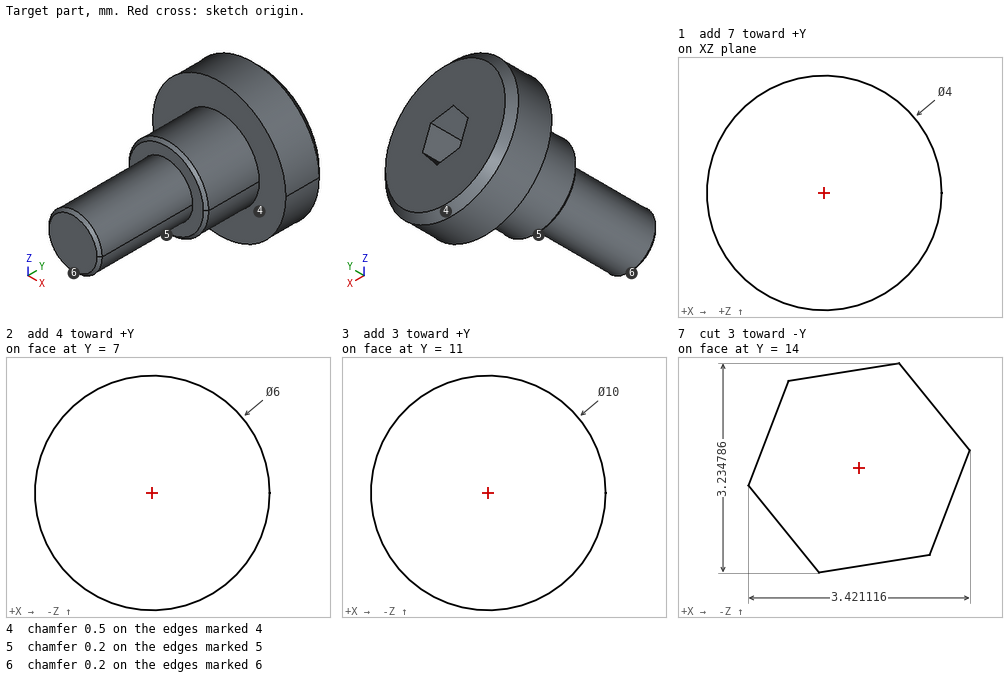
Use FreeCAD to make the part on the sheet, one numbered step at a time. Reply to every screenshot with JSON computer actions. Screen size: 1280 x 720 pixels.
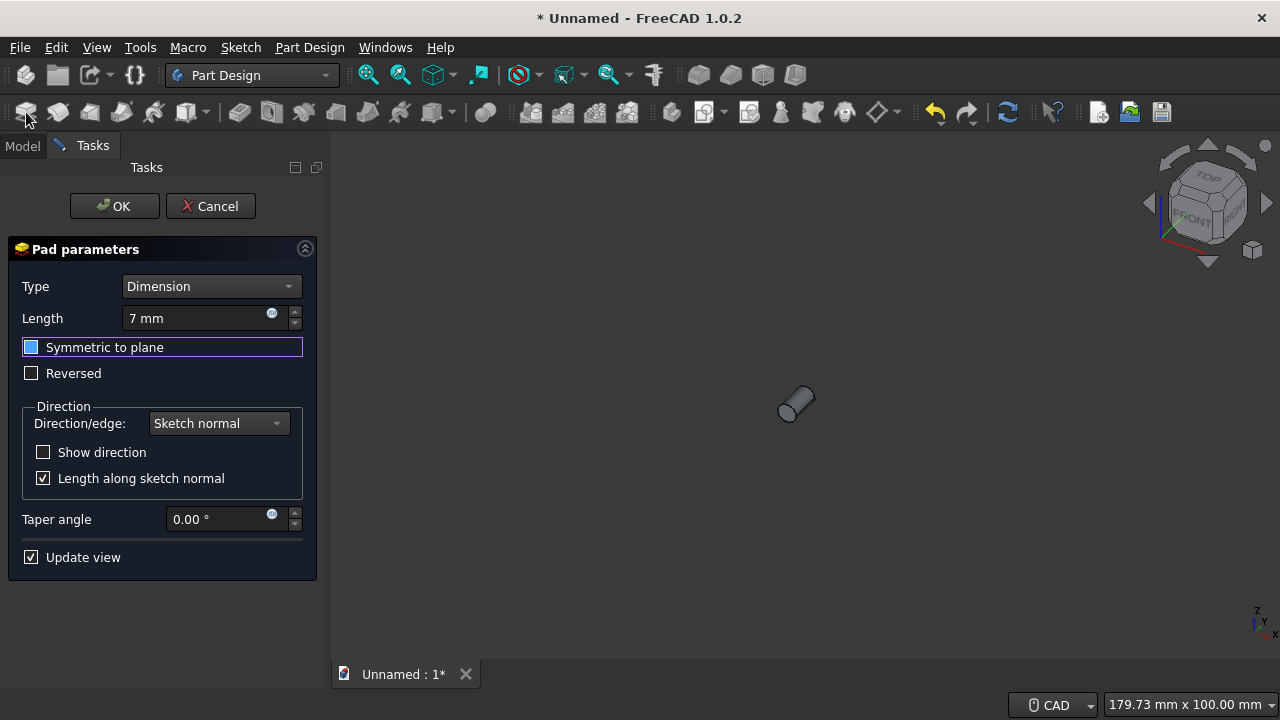
{"action": "left_click", "coordinate": [30, 373]}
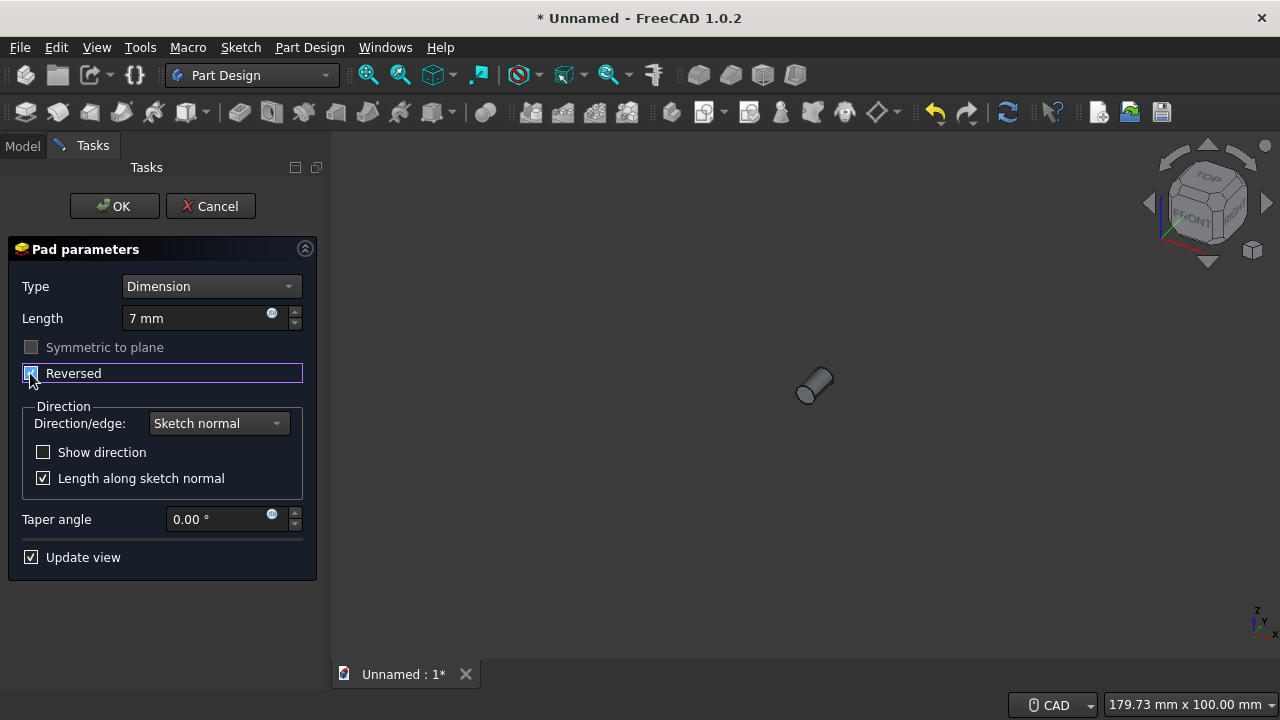
{"action": "left_click", "coordinate": [115, 206]}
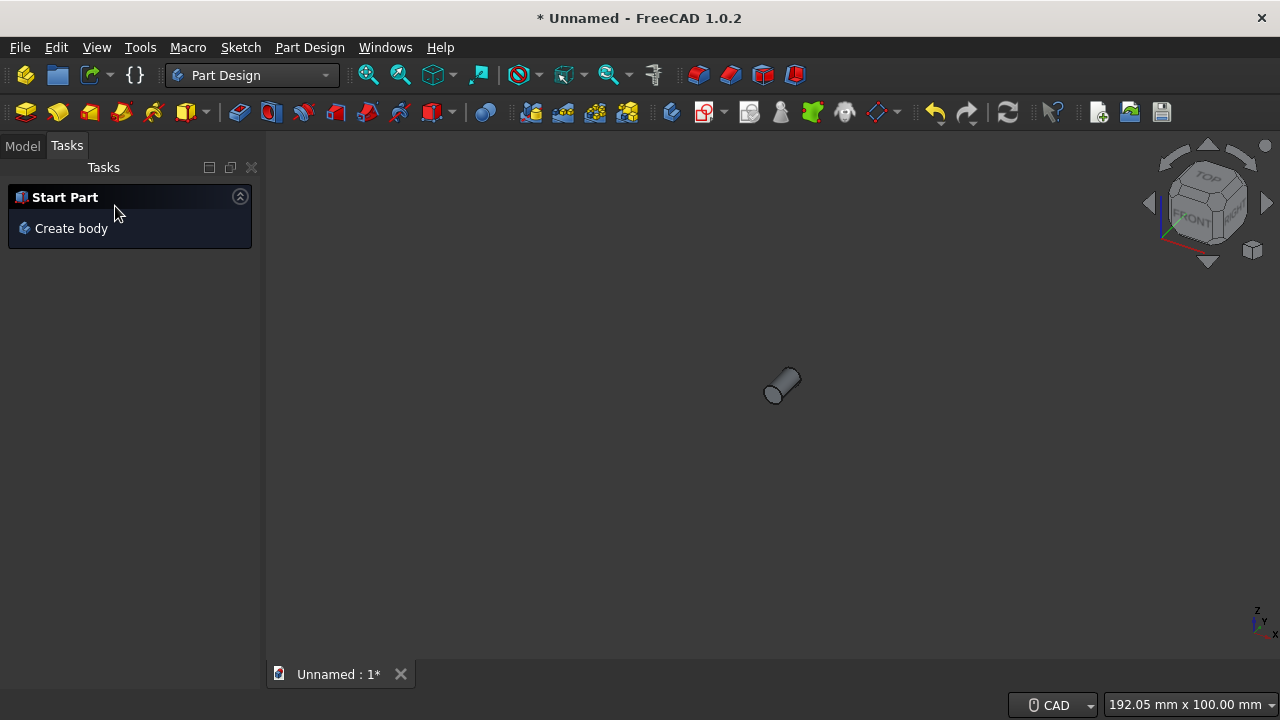
{"action": "key", "text": "v f"}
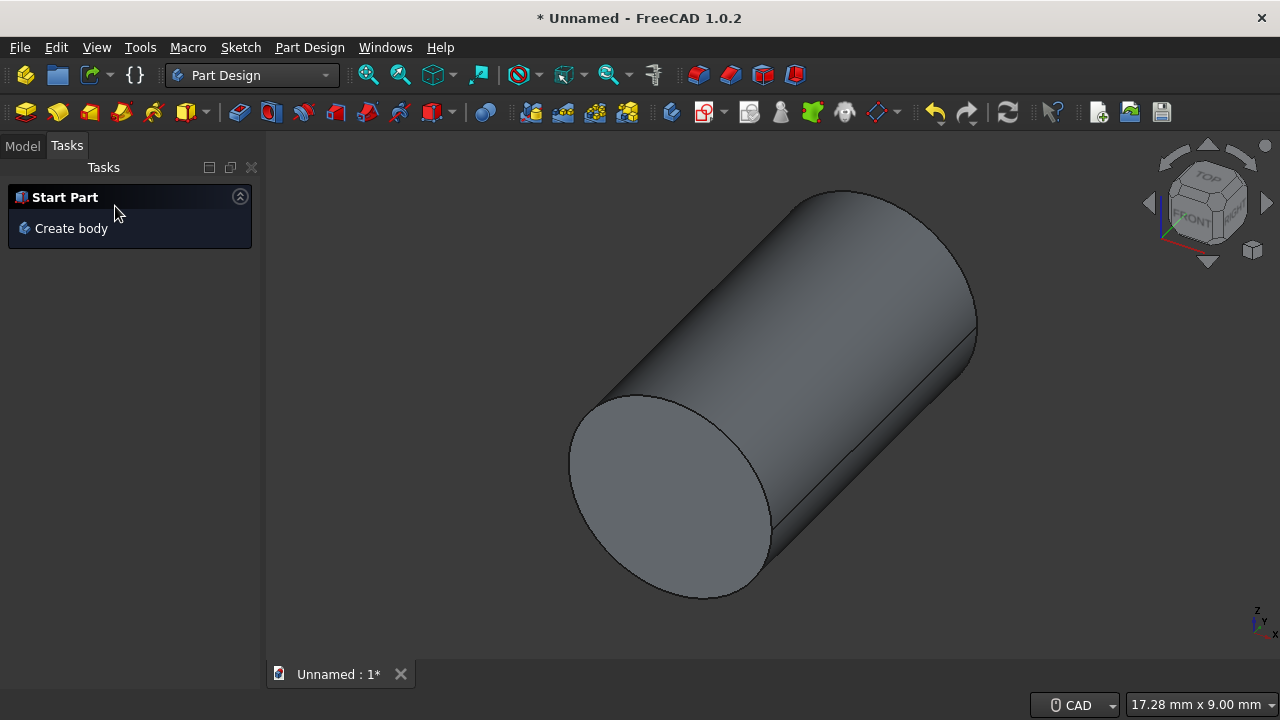
{"action": "key", "text": "4"}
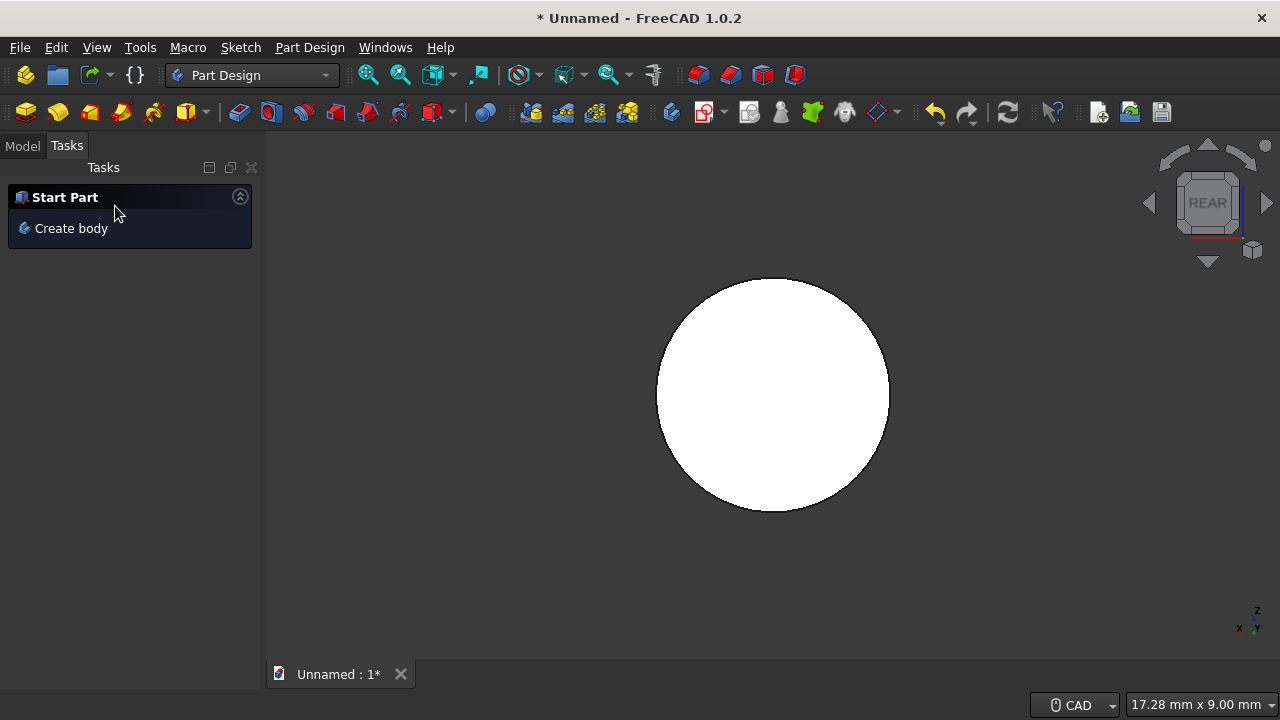
{"action": "left_click", "coordinate": [370, 76]}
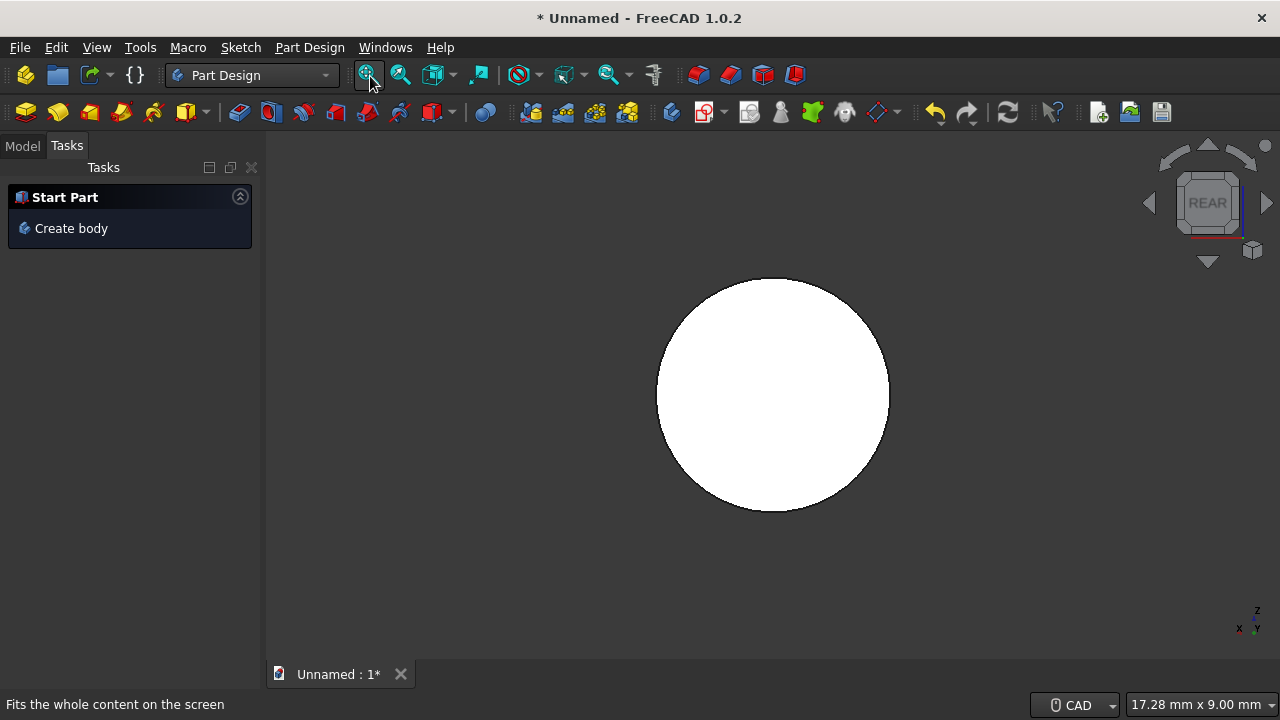
{"action": "left_click", "coordinate": [773, 394]}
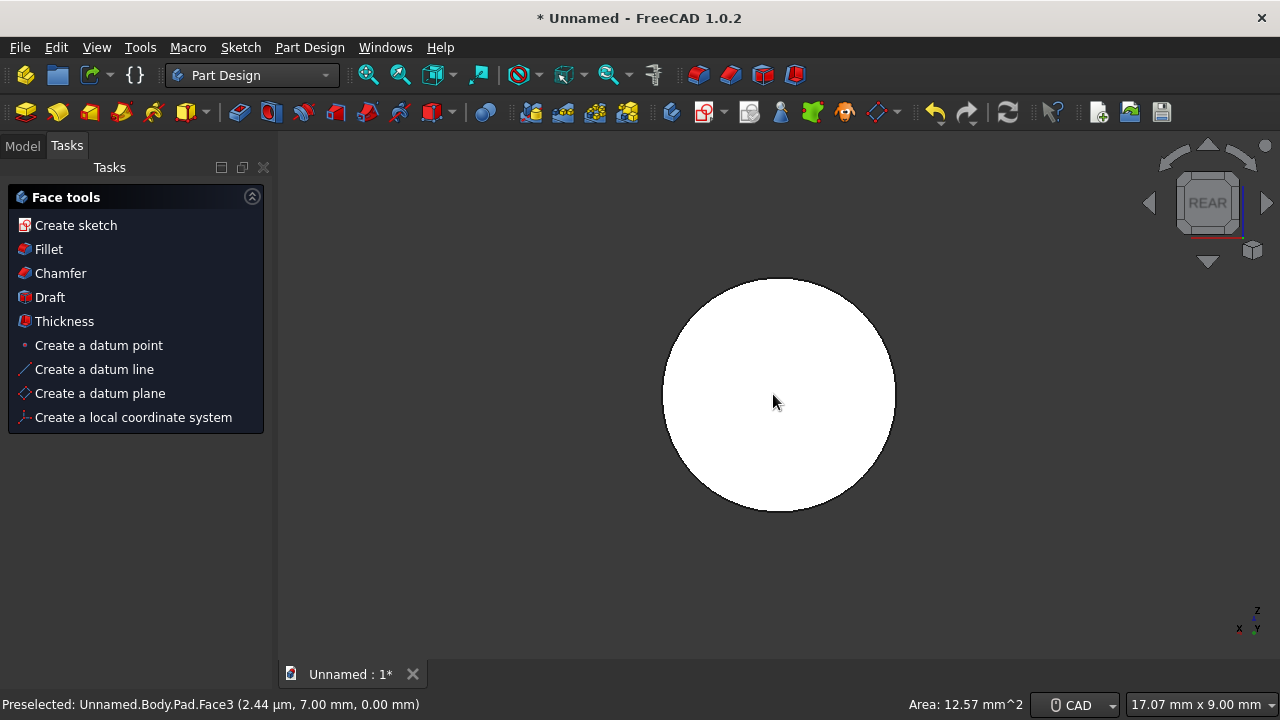
{"action": "left_click", "coordinate": [704, 112]}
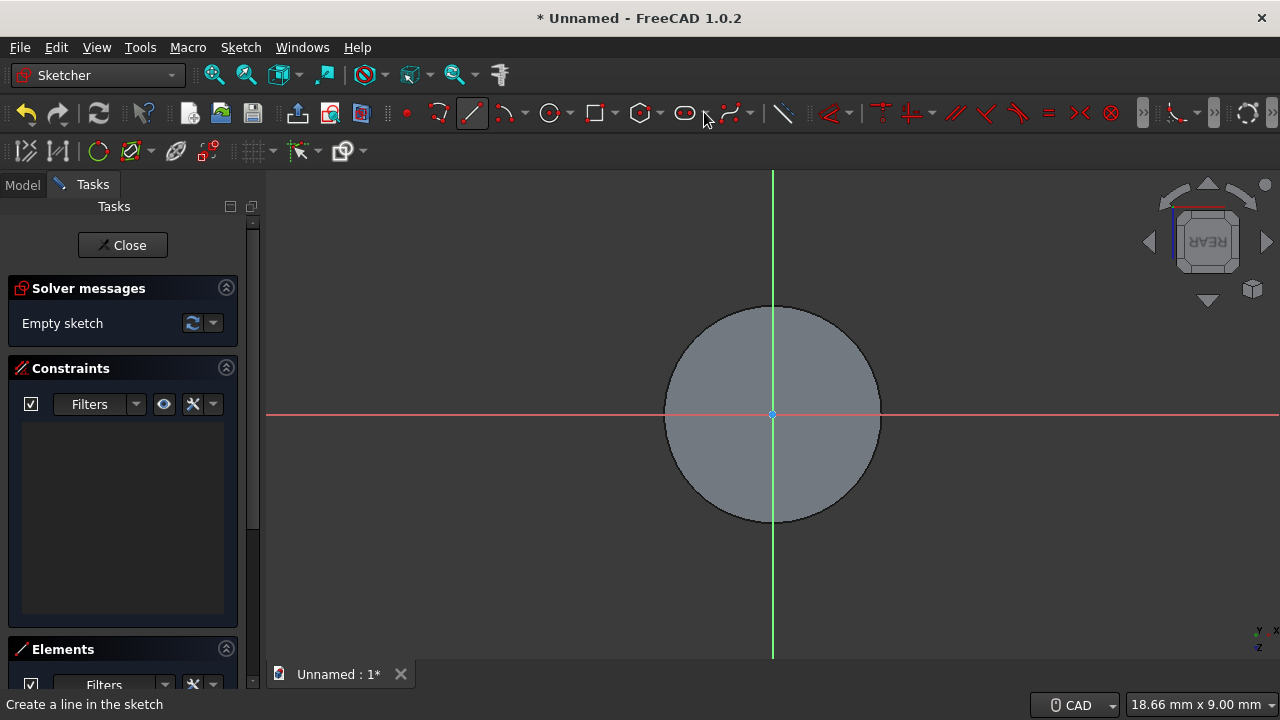
{"action": "key", "text": "g c"}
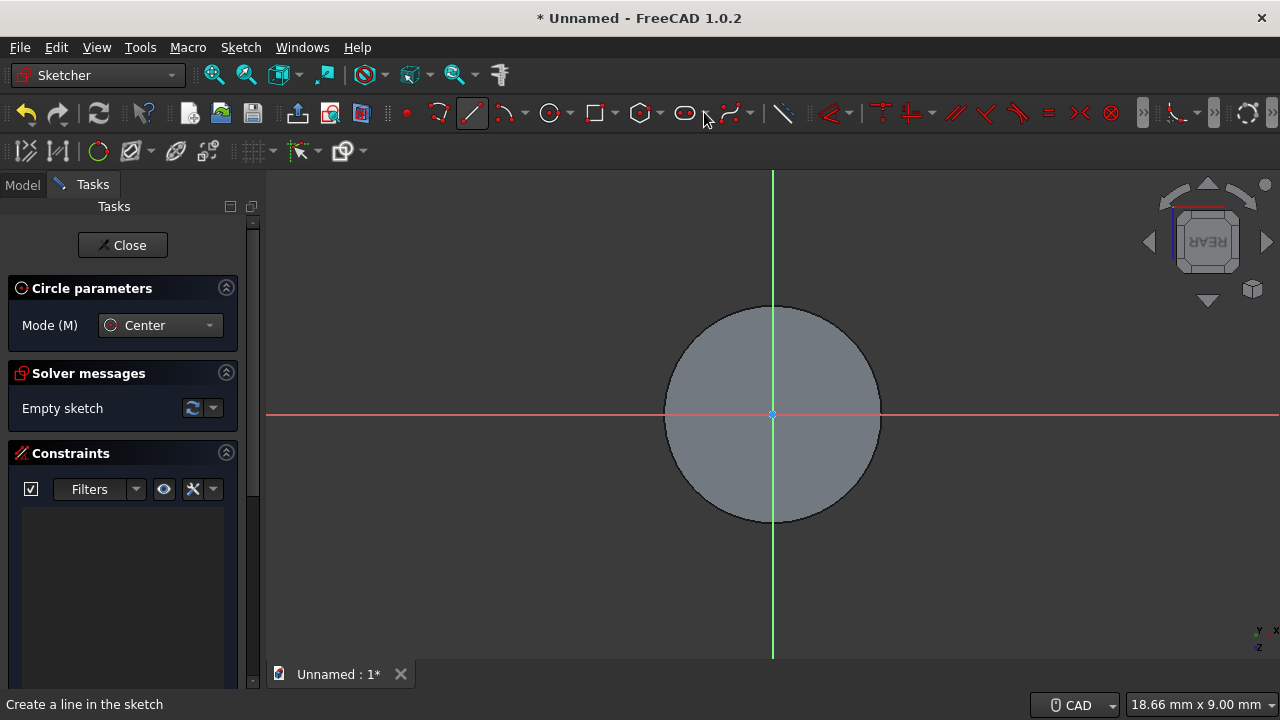
{"action": "left_click", "coordinate": [773, 414]}
{"action": "mouse_move", "coordinate": [888, 299]}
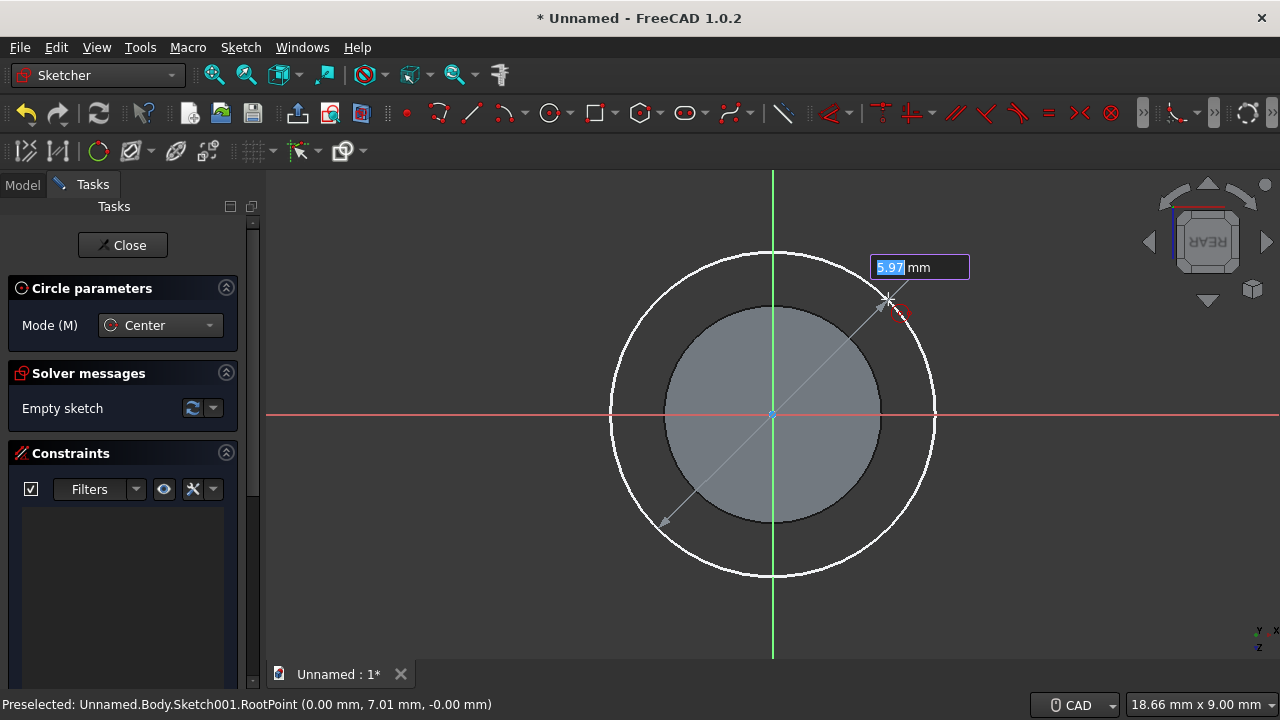
{"action": "type", "text": "6"}
{"action": "key", "text": "Return"}
{"action": "key", "text": "Escape"}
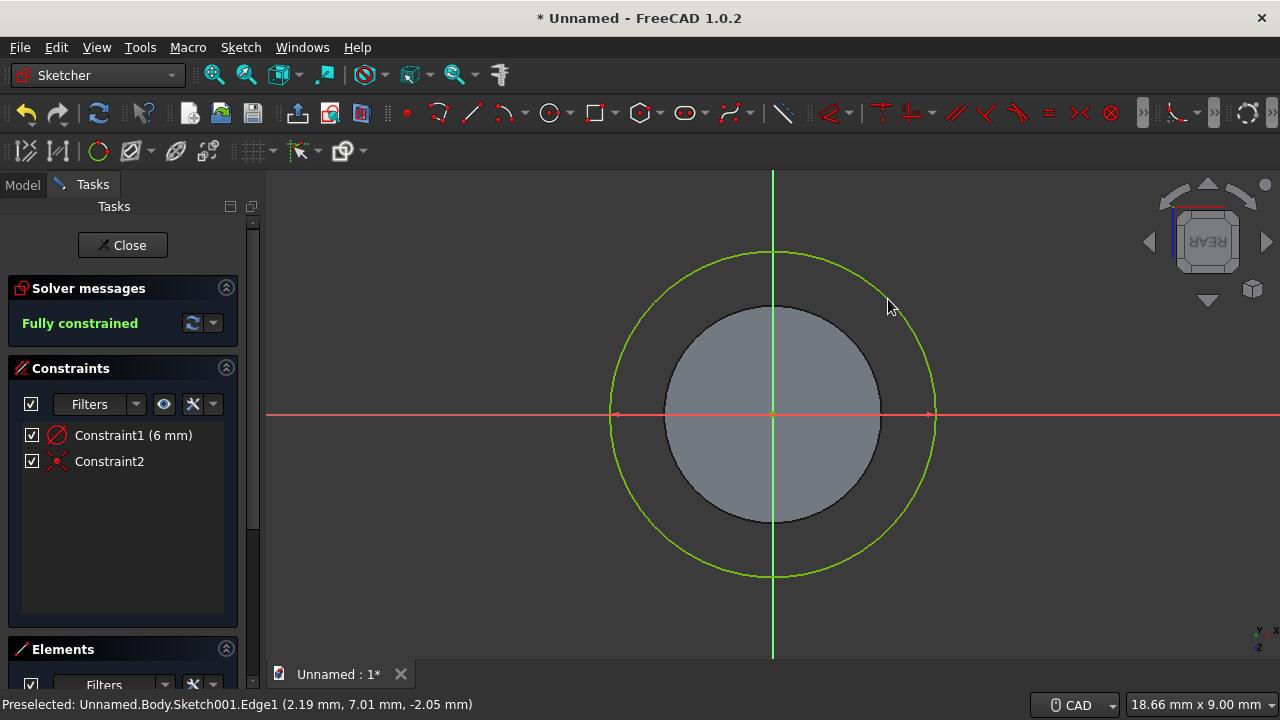
{"action": "left_click", "coordinate": [123, 245]}